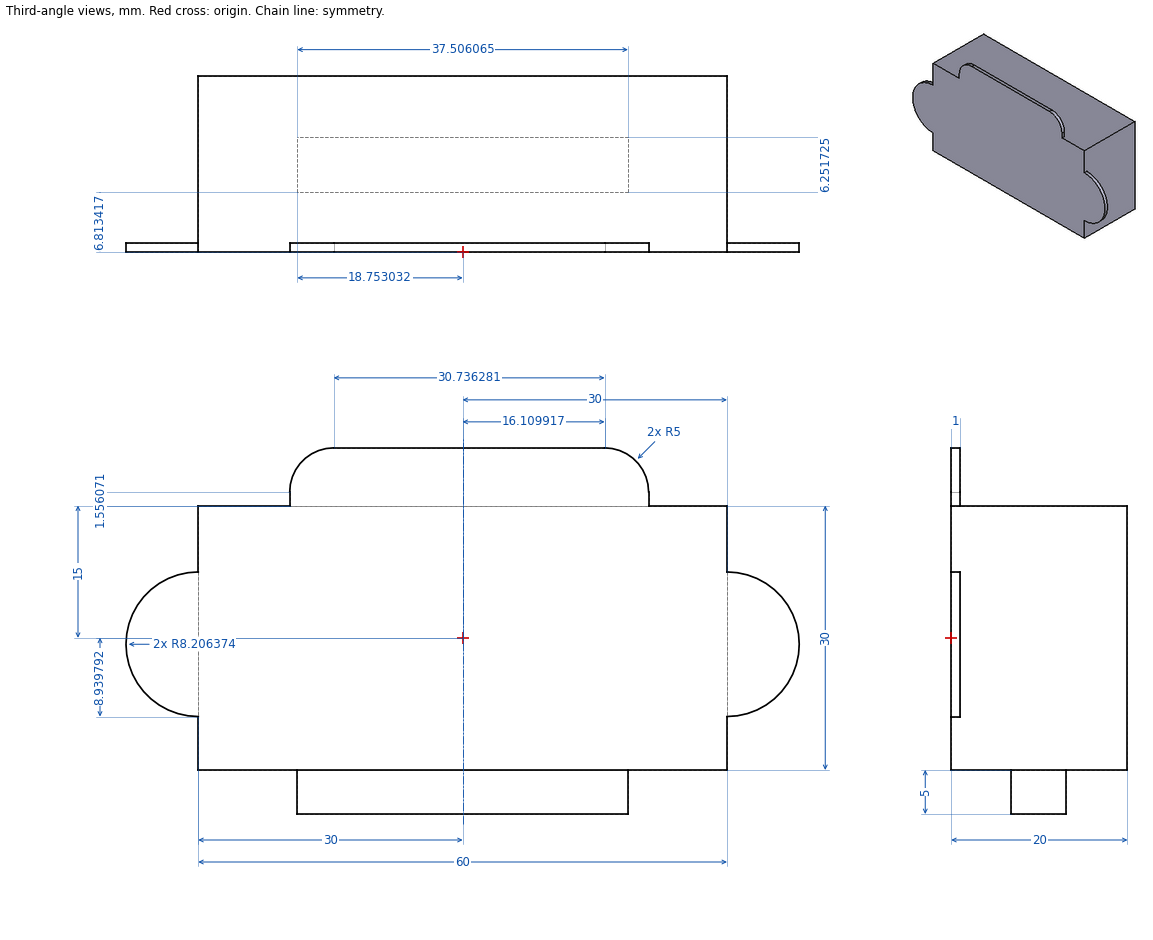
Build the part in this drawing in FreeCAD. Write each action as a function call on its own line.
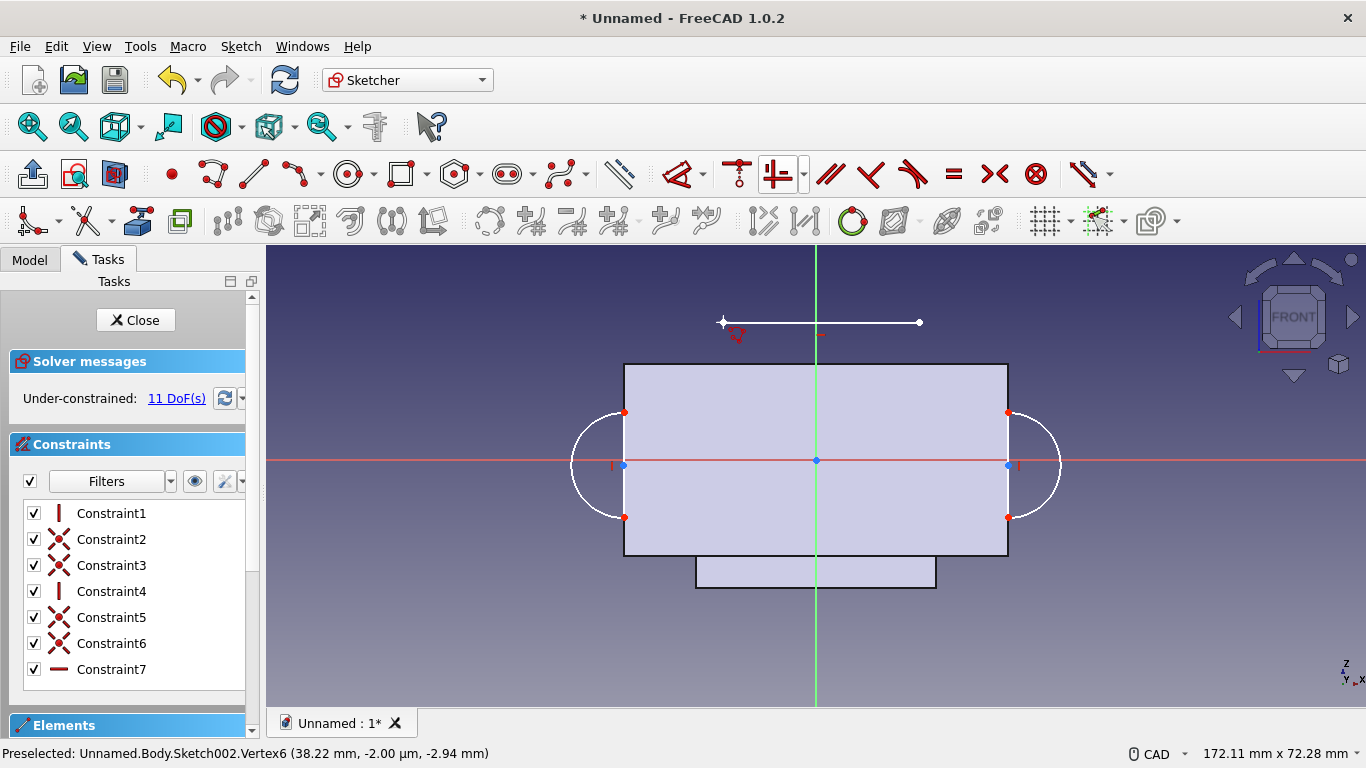
click(691, 354)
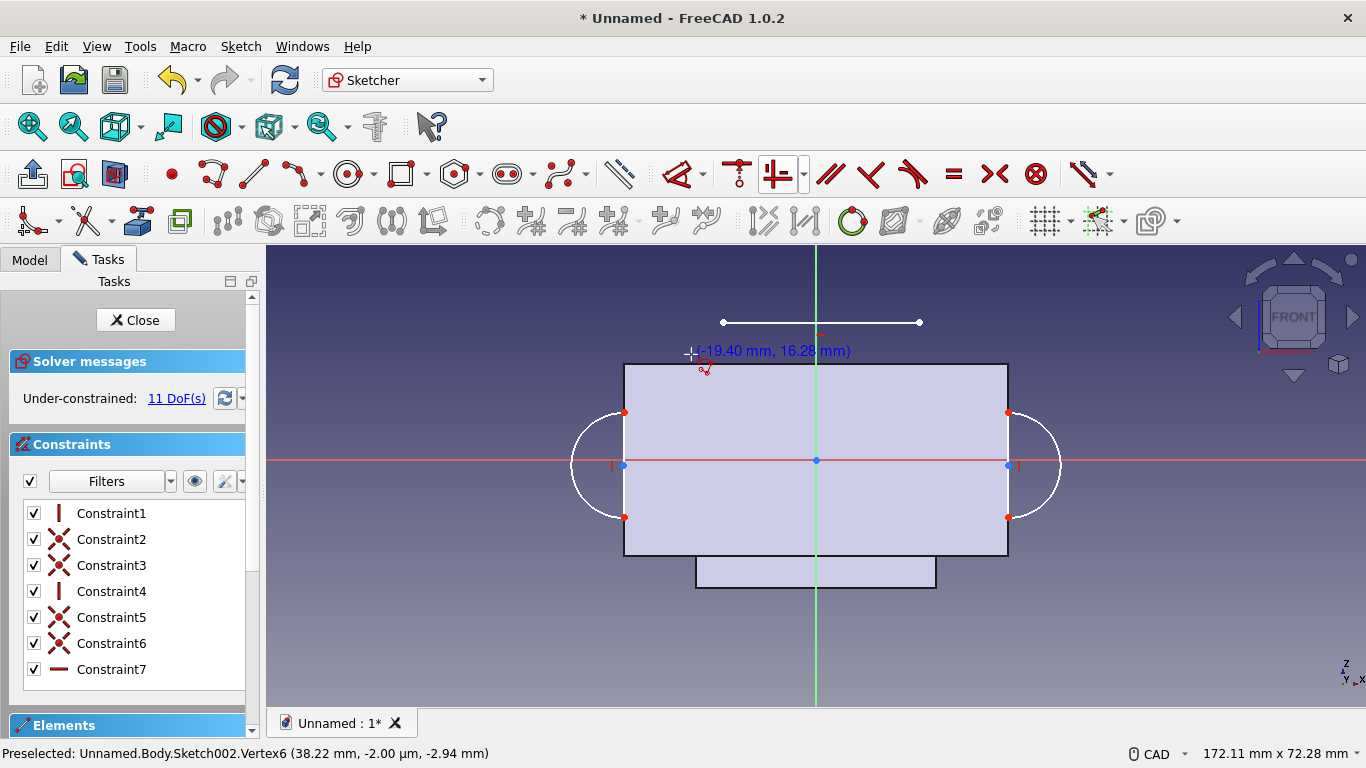
scroll(691, 364, up, 3)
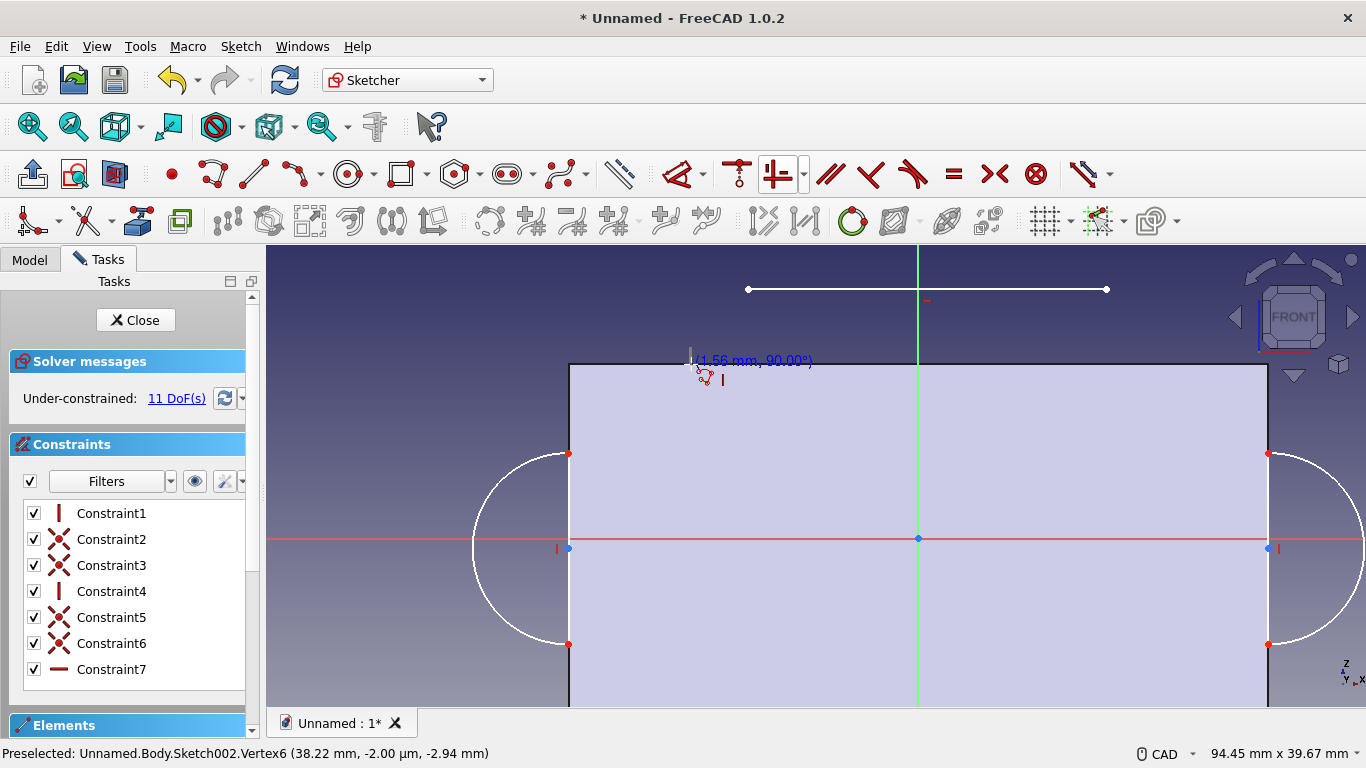
click(691, 364)
click(1164, 364)
click(1164, 346)
right_click(1164, 346)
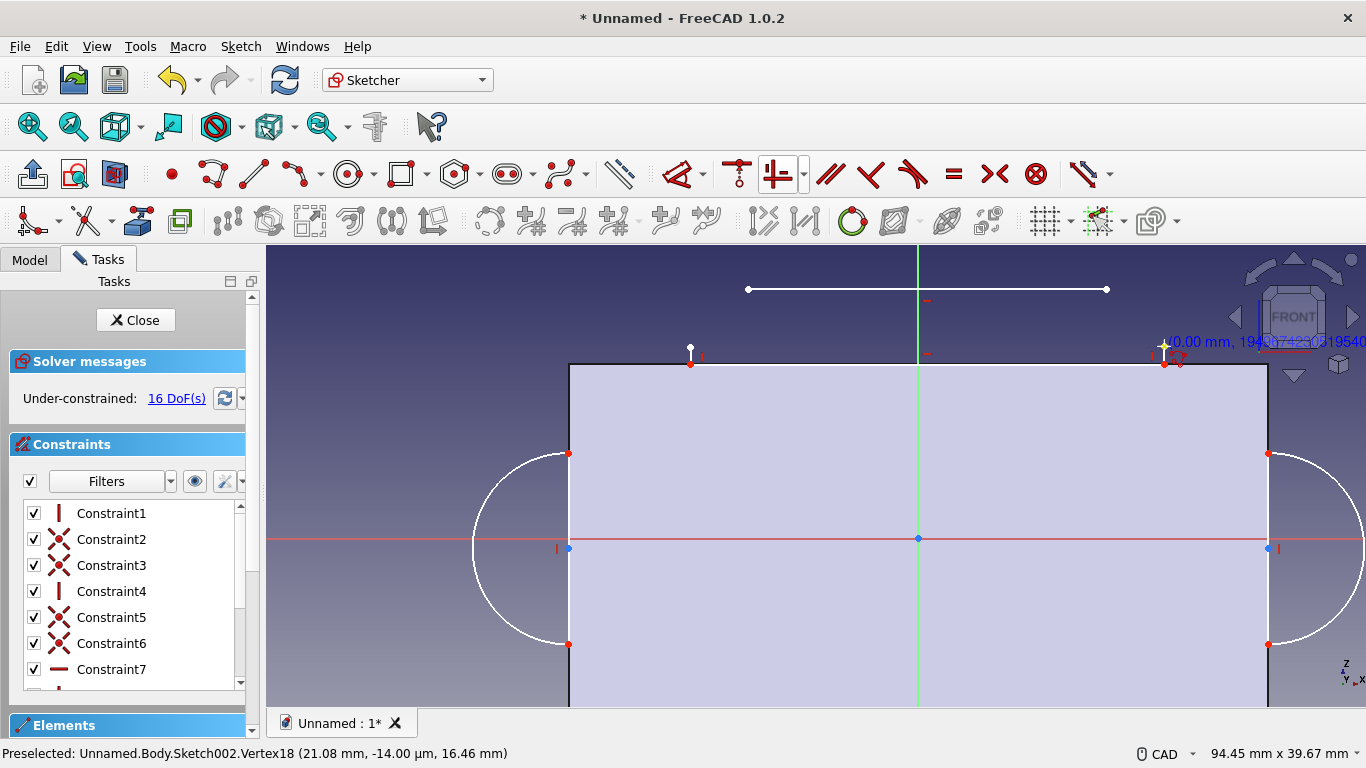
click(294, 174)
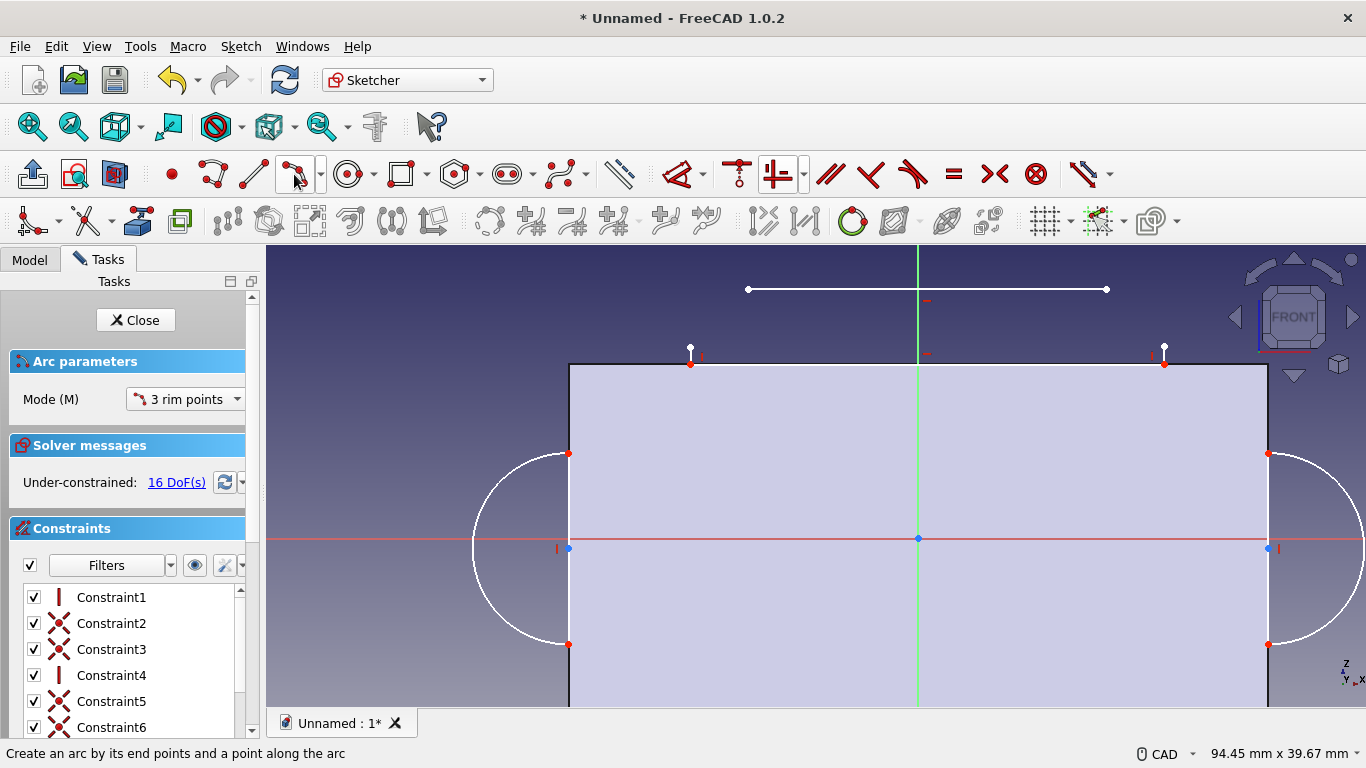
click(749, 289)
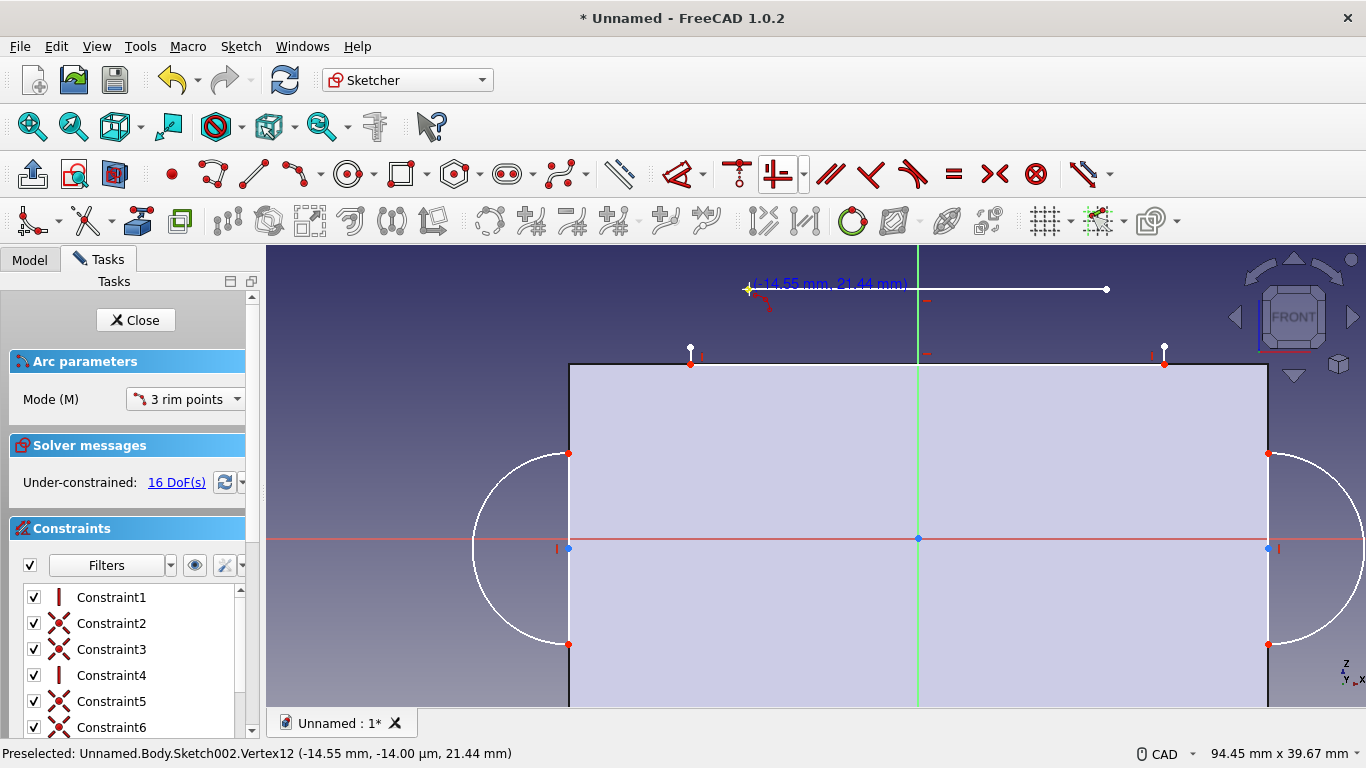
scroll(690, 346, up, 3)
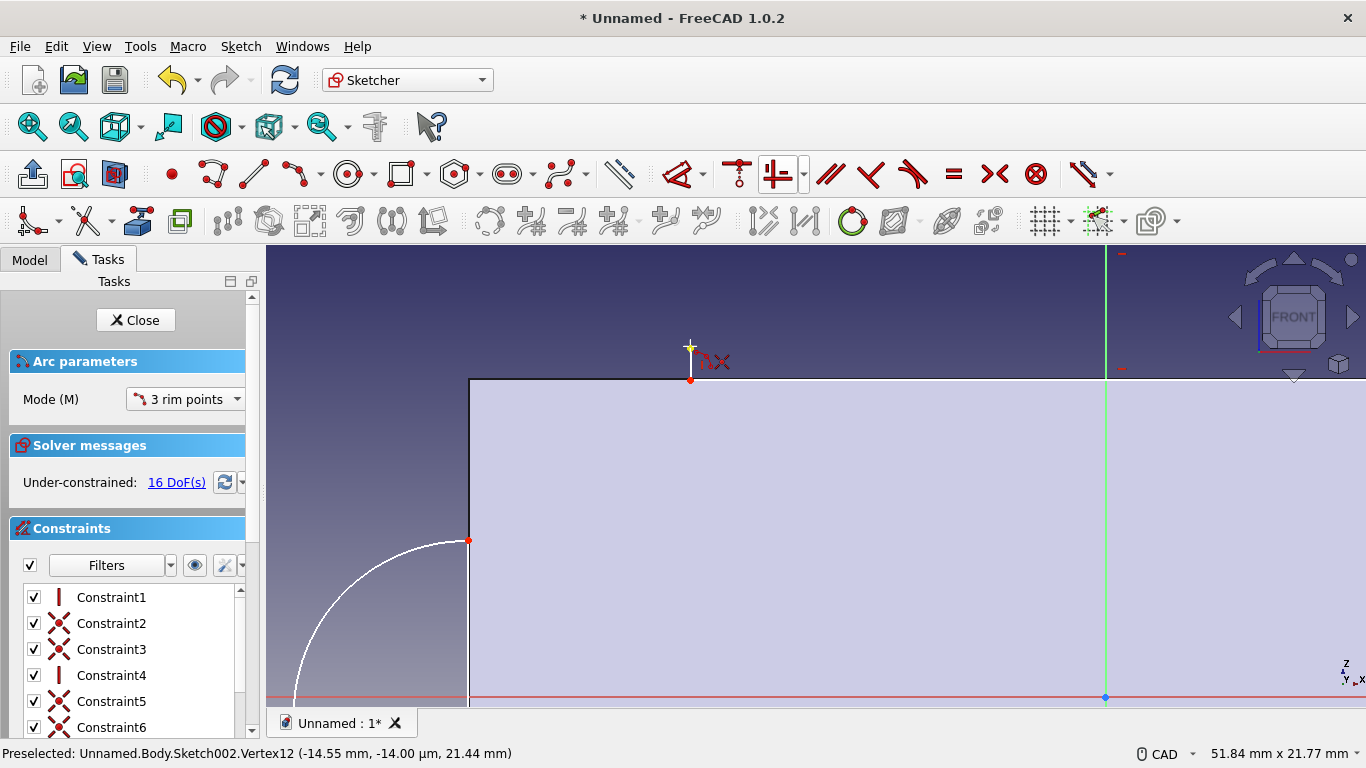
click(691, 348)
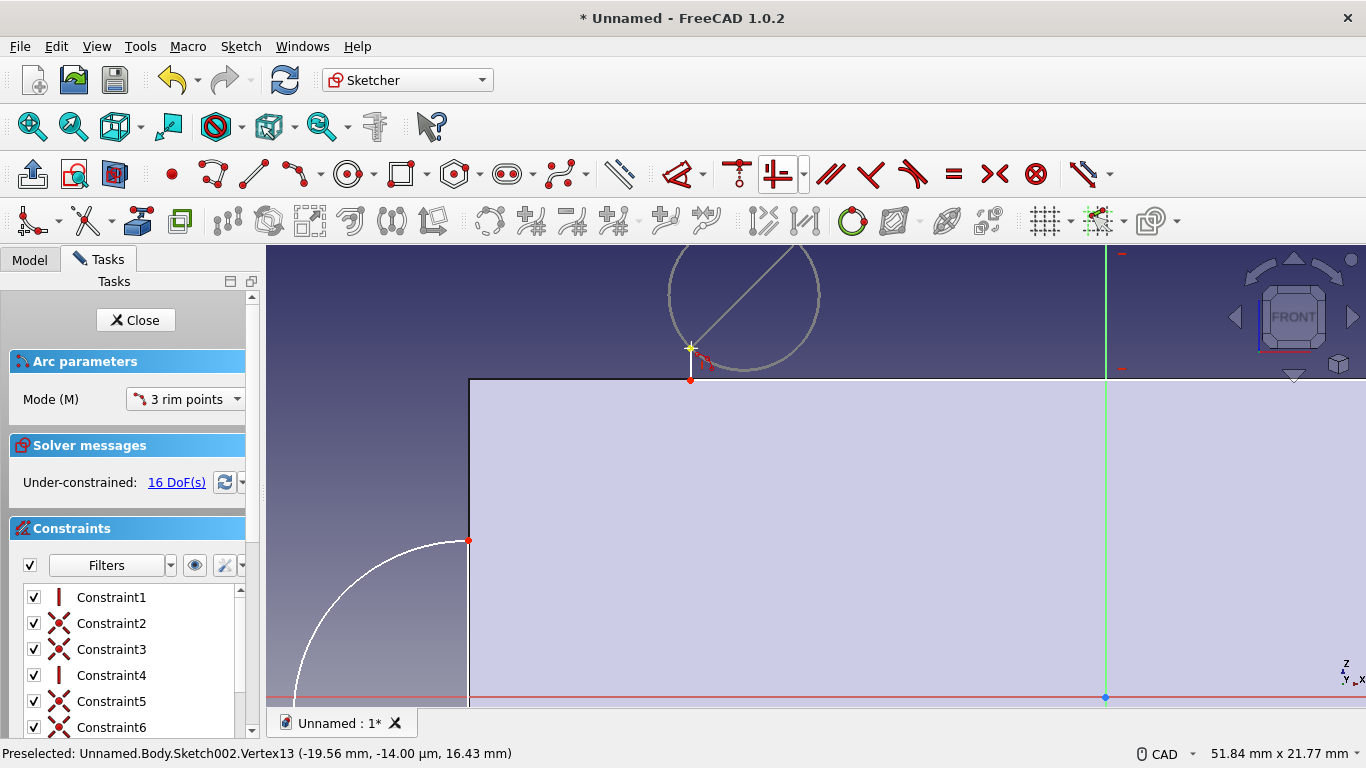
scroll(539, 425, down, 5)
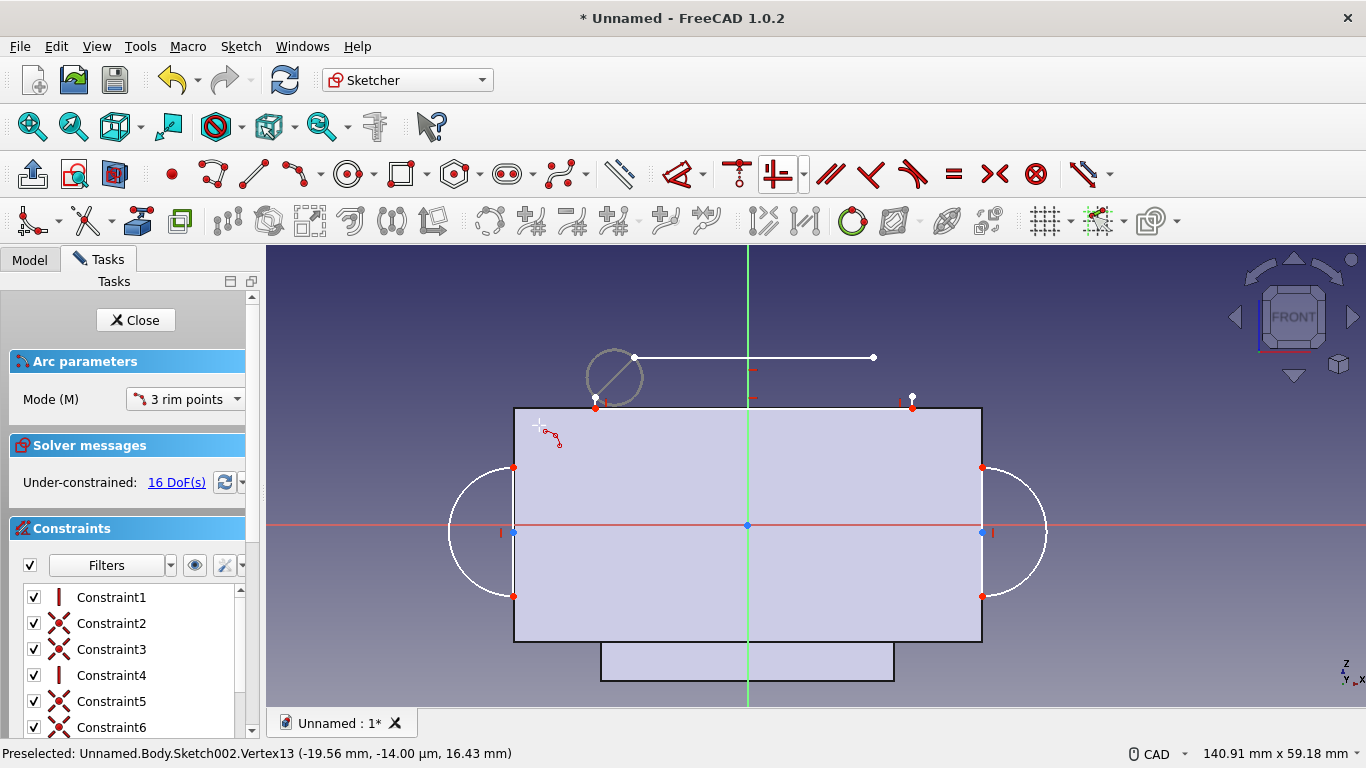
scroll(606, 368, up, 2)